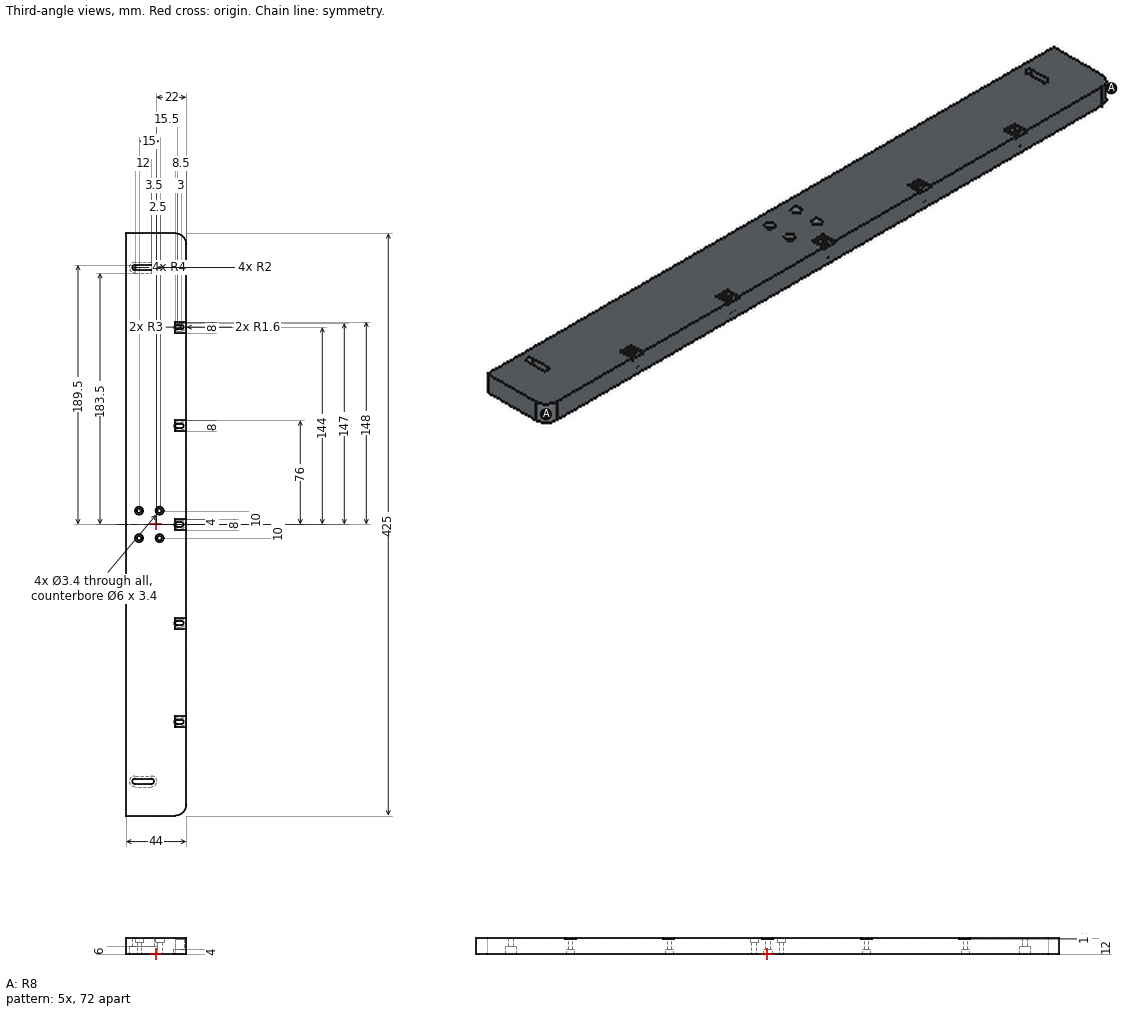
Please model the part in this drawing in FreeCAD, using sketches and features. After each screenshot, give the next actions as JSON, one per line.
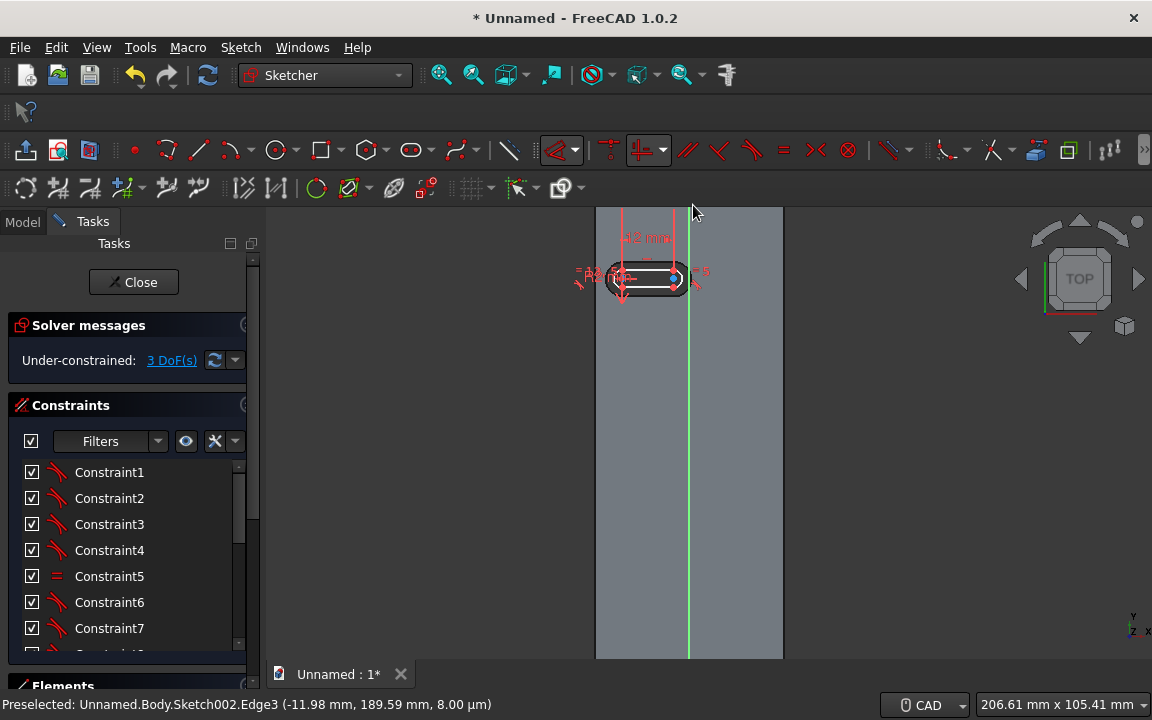
{"action": "scroll", "coordinate": [638, 304], "scroll_direction": "down", "scroll_amount": 9}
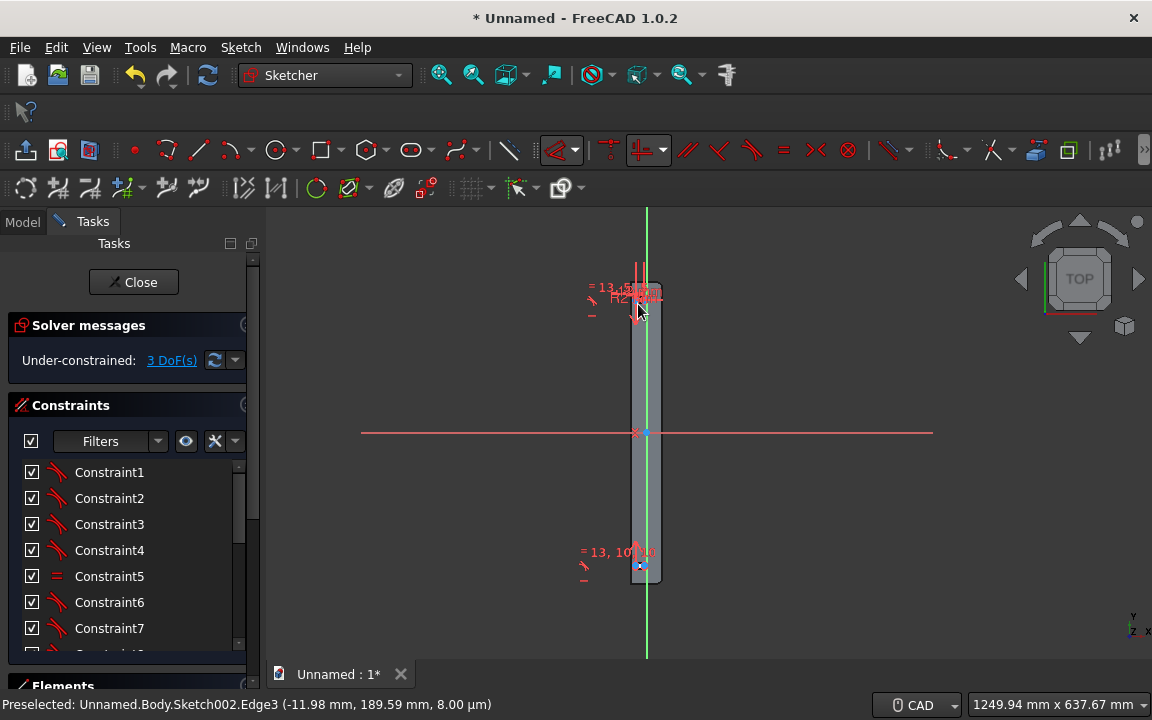
{"action": "scroll", "coordinate": [638, 565], "scroll_direction": "up", "scroll_amount": 9}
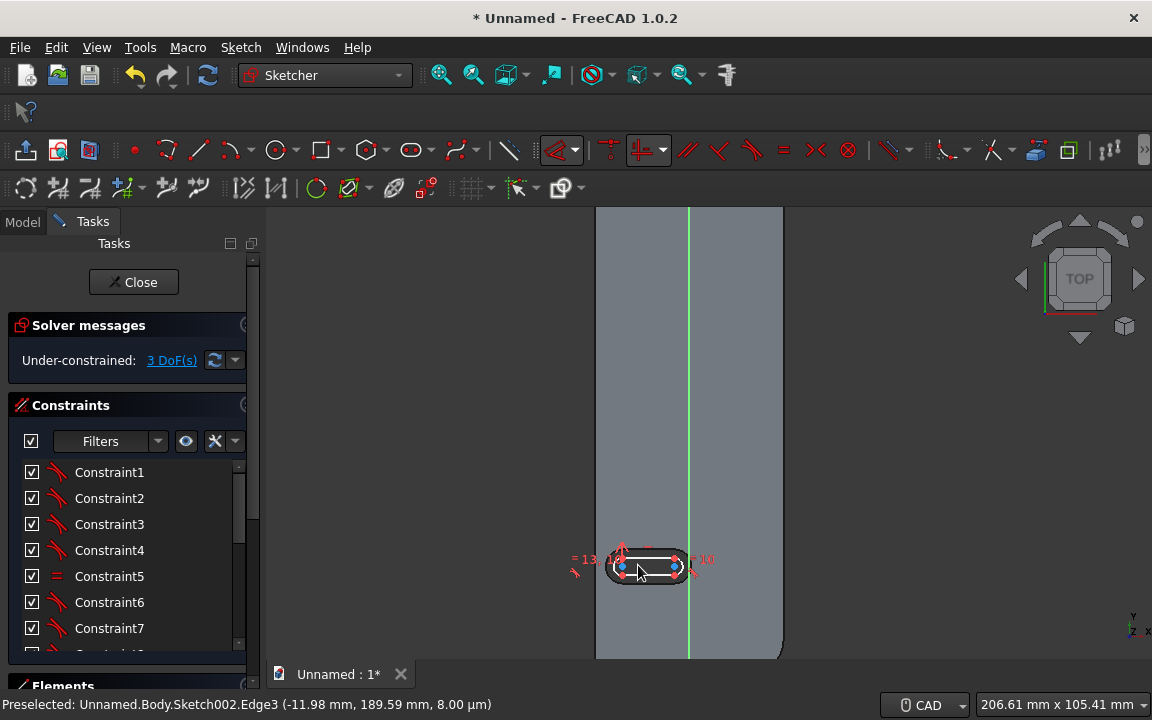
{"action": "left_click", "coordinate": [638, 558]}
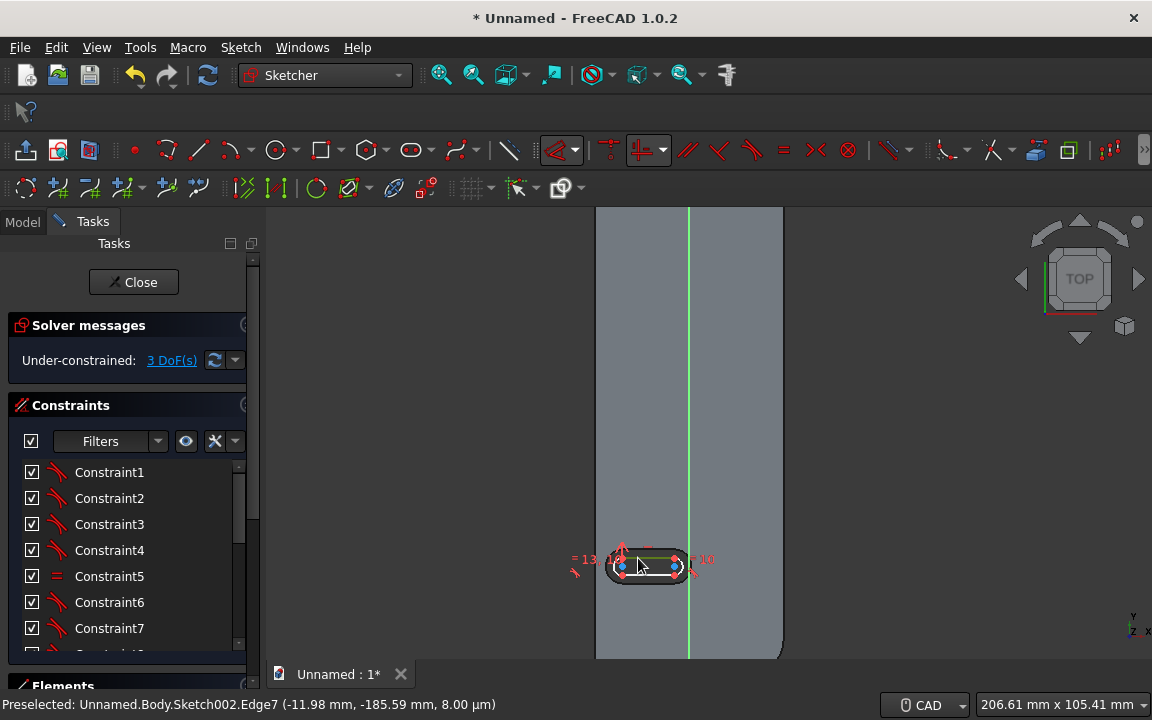
{"action": "key", "text": "l"}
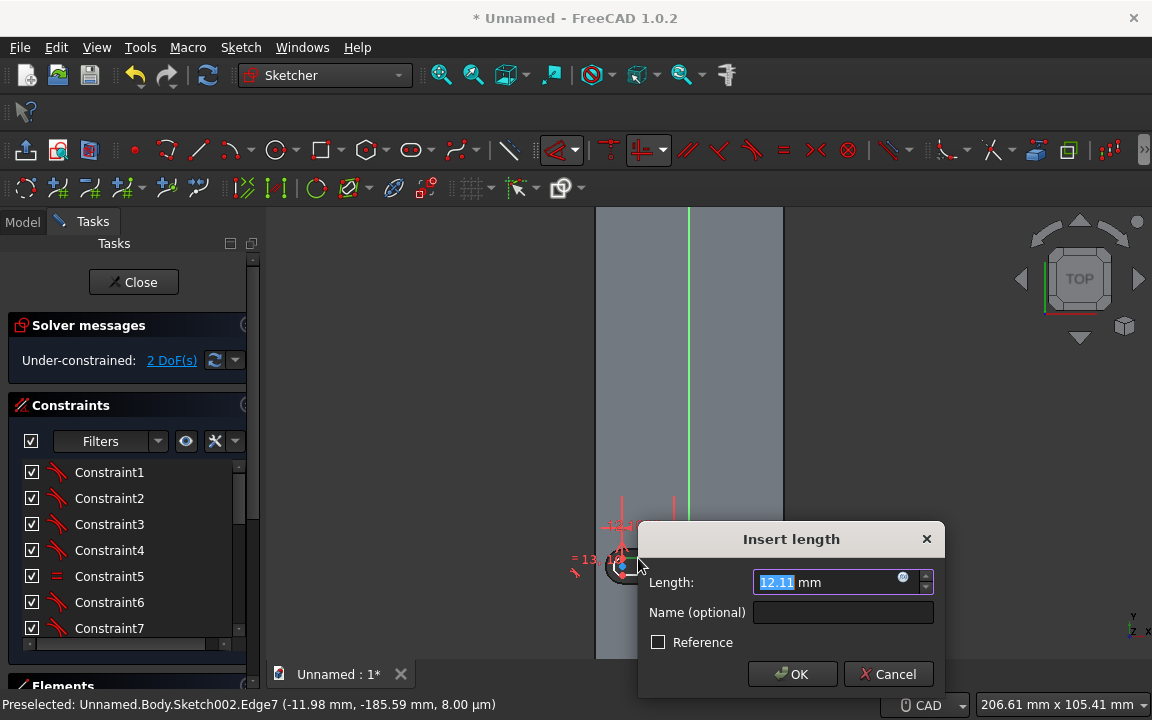
{"action": "type", "text": "12"}
{"action": "key", "text": "Return"}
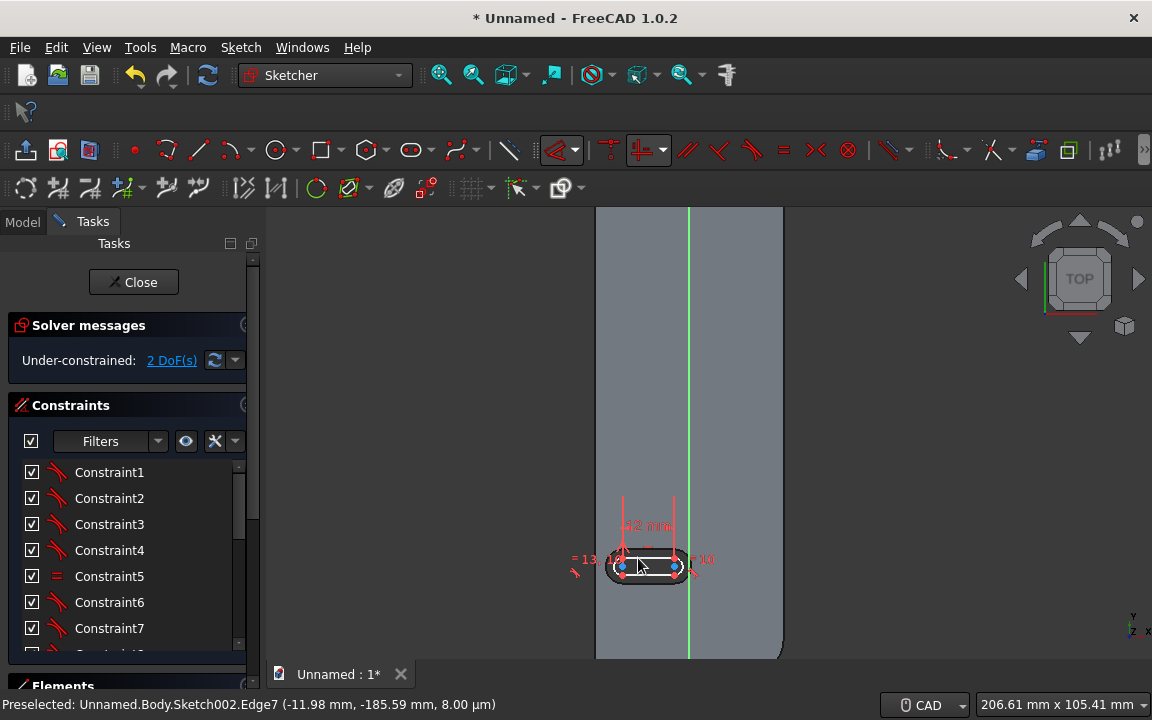
{"action": "scroll", "coordinate": [638, 566], "scroll_direction": "down", "scroll_amount": 9}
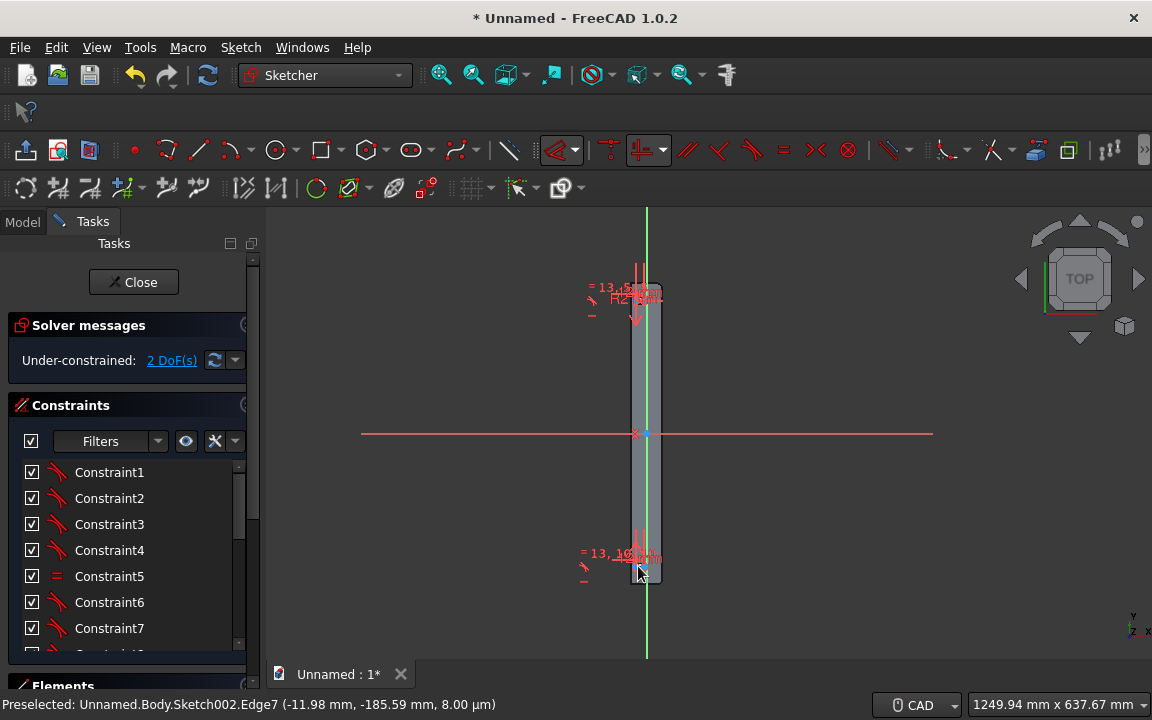
{"action": "scroll", "coordinate": [644, 302], "scroll_direction": "up", "scroll_amount": 14}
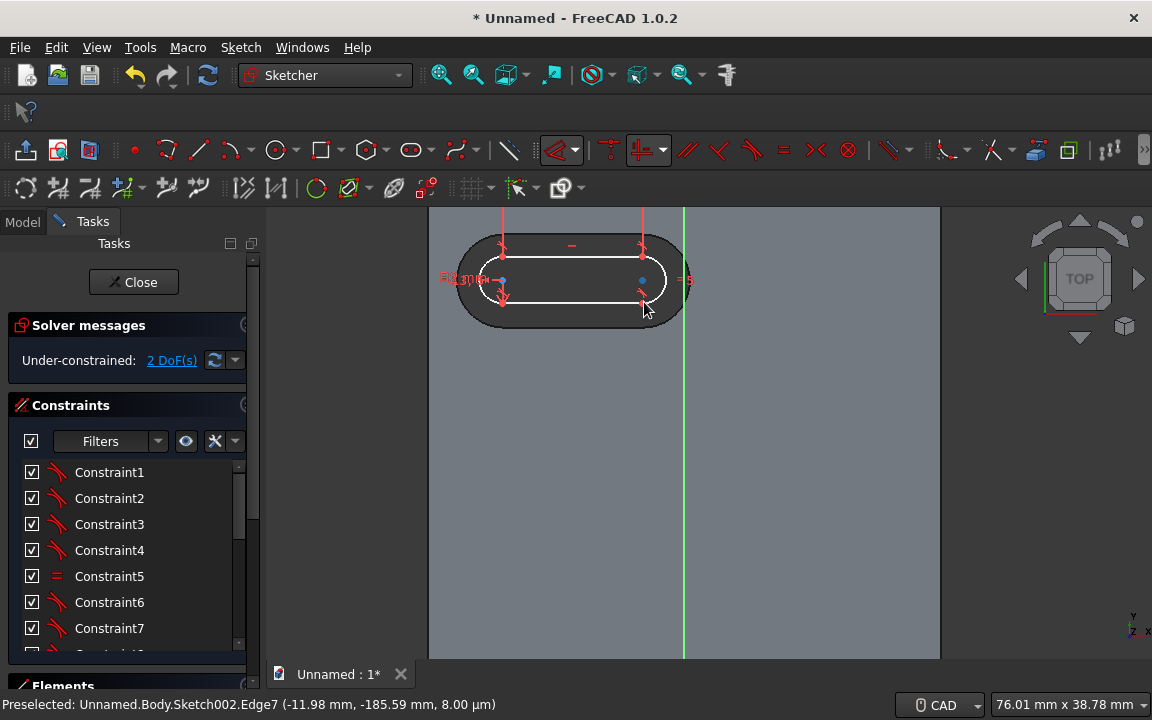
{"action": "left_click", "coordinate": [643, 303]}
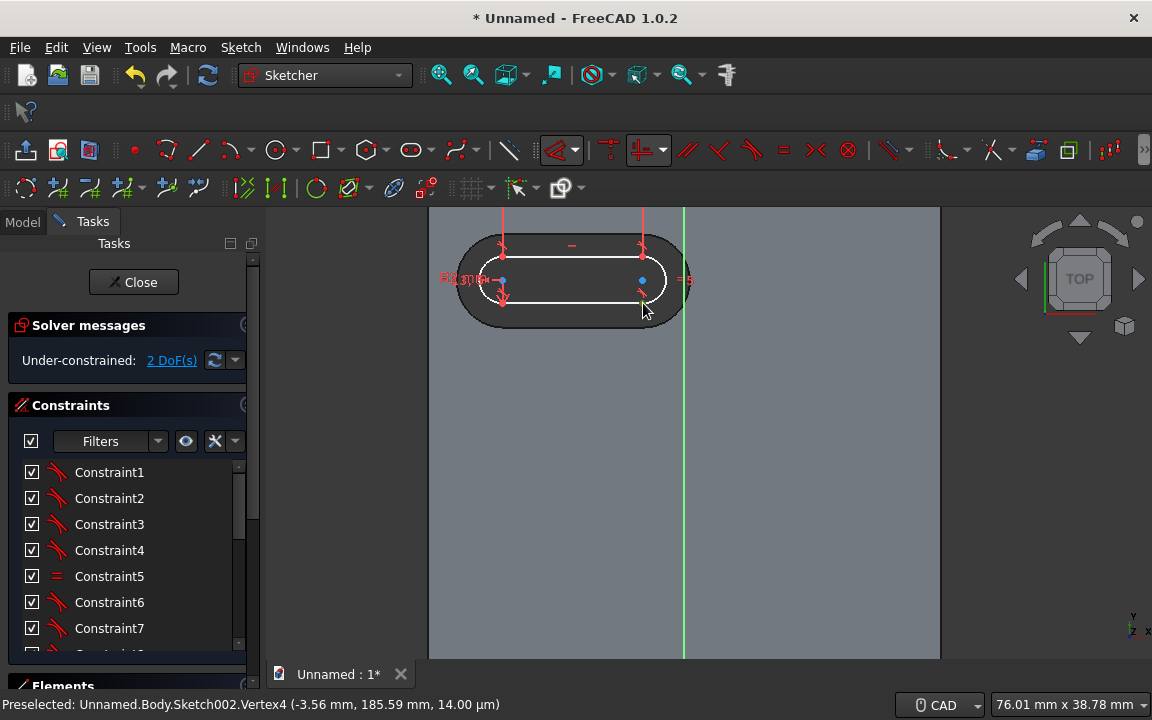
{"action": "left_click", "coordinate": [578, 150]}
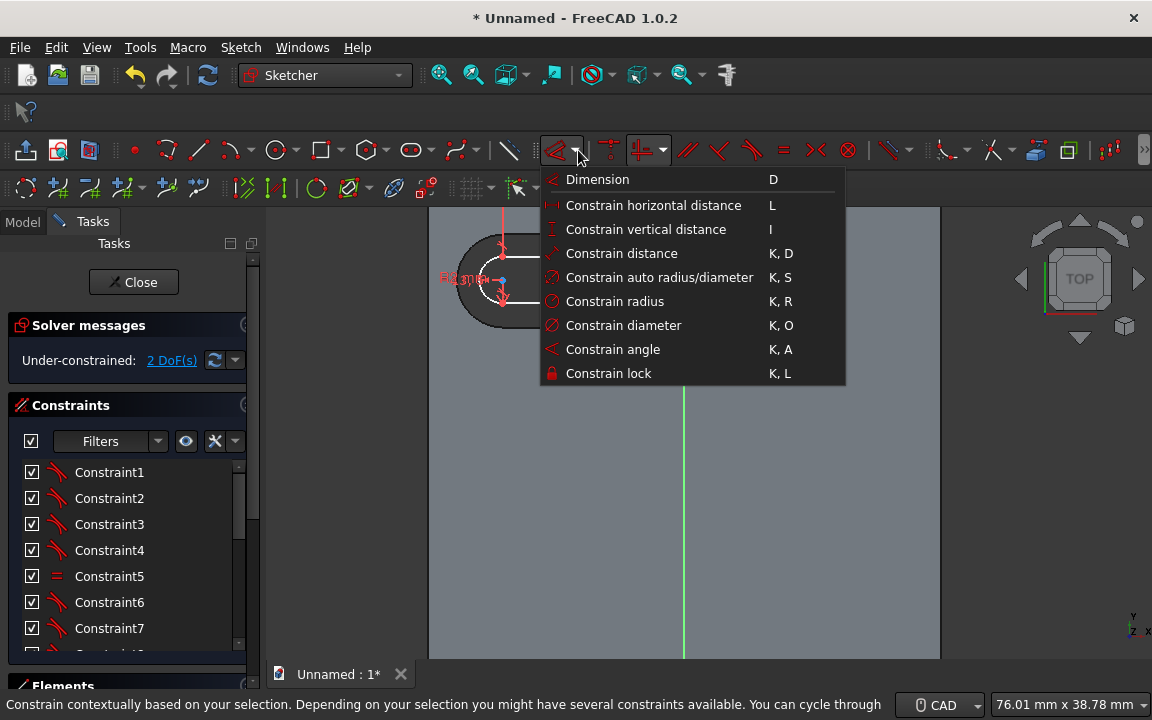
{"action": "left_click", "coordinate": [693, 205]}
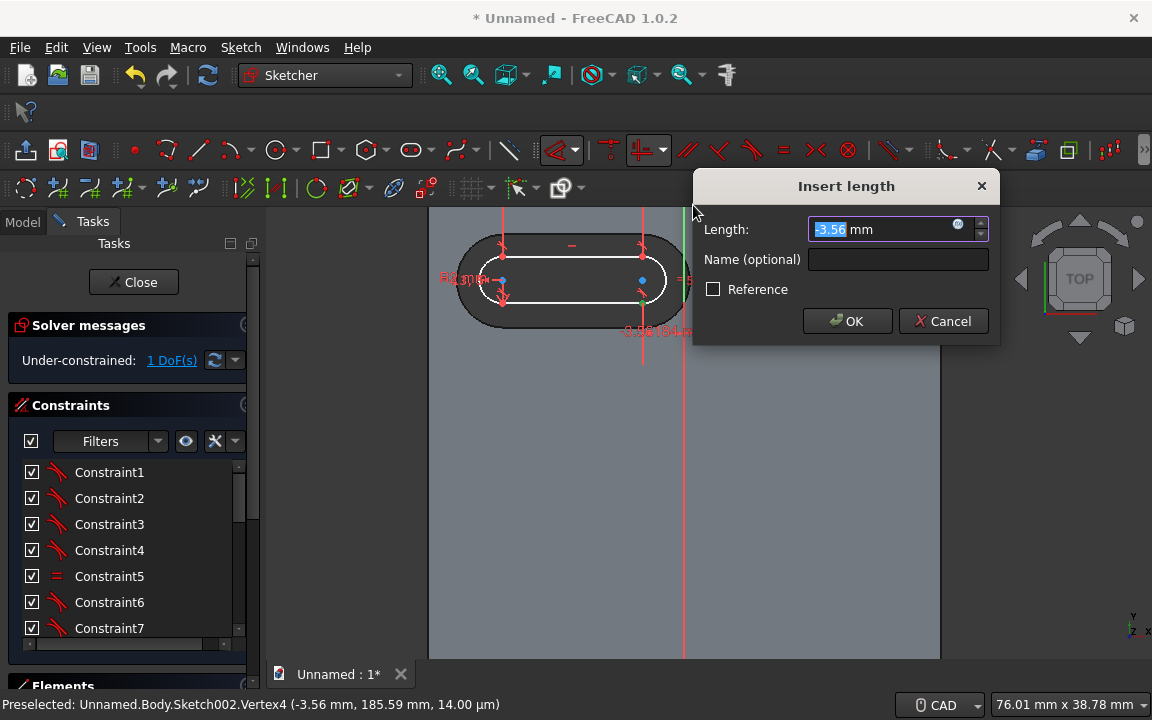
{"action": "type", "text": "-3.5"}
{"action": "key", "text": "Return"}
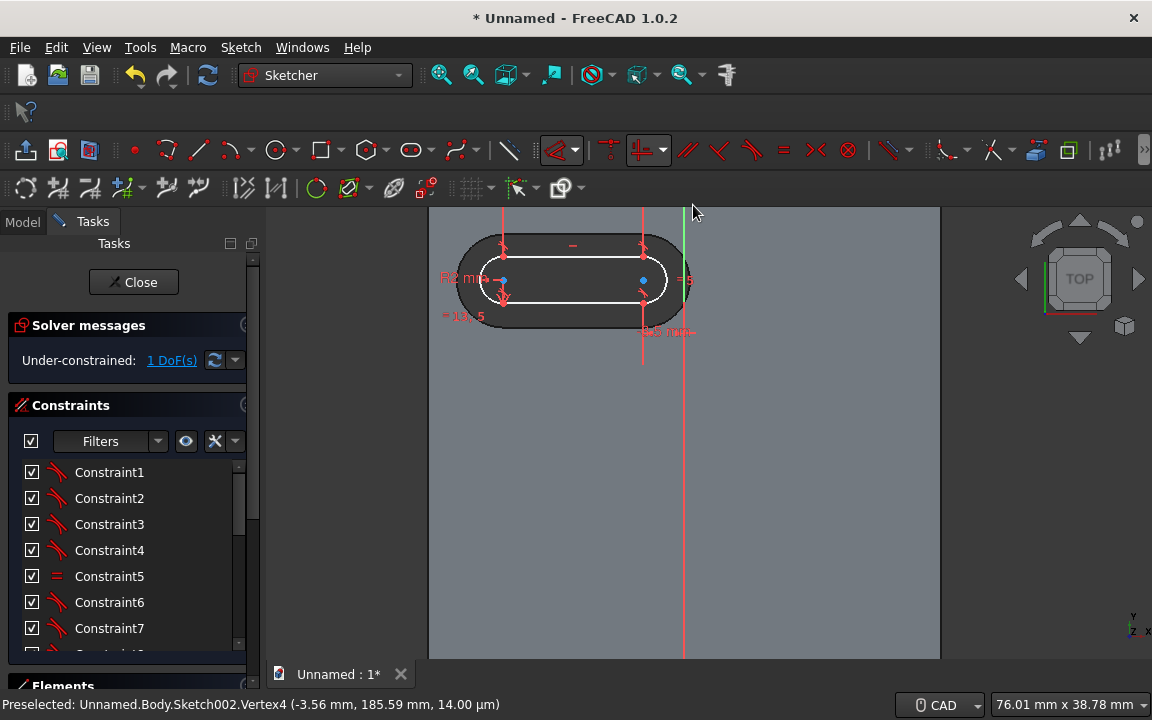
{"action": "left_click", "coordinate": [503, 257]}